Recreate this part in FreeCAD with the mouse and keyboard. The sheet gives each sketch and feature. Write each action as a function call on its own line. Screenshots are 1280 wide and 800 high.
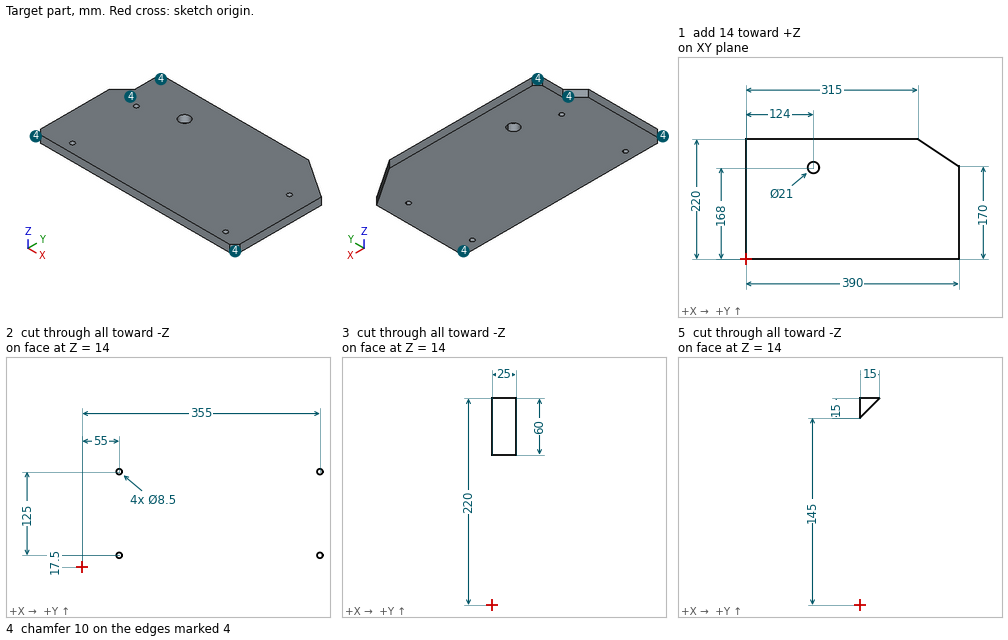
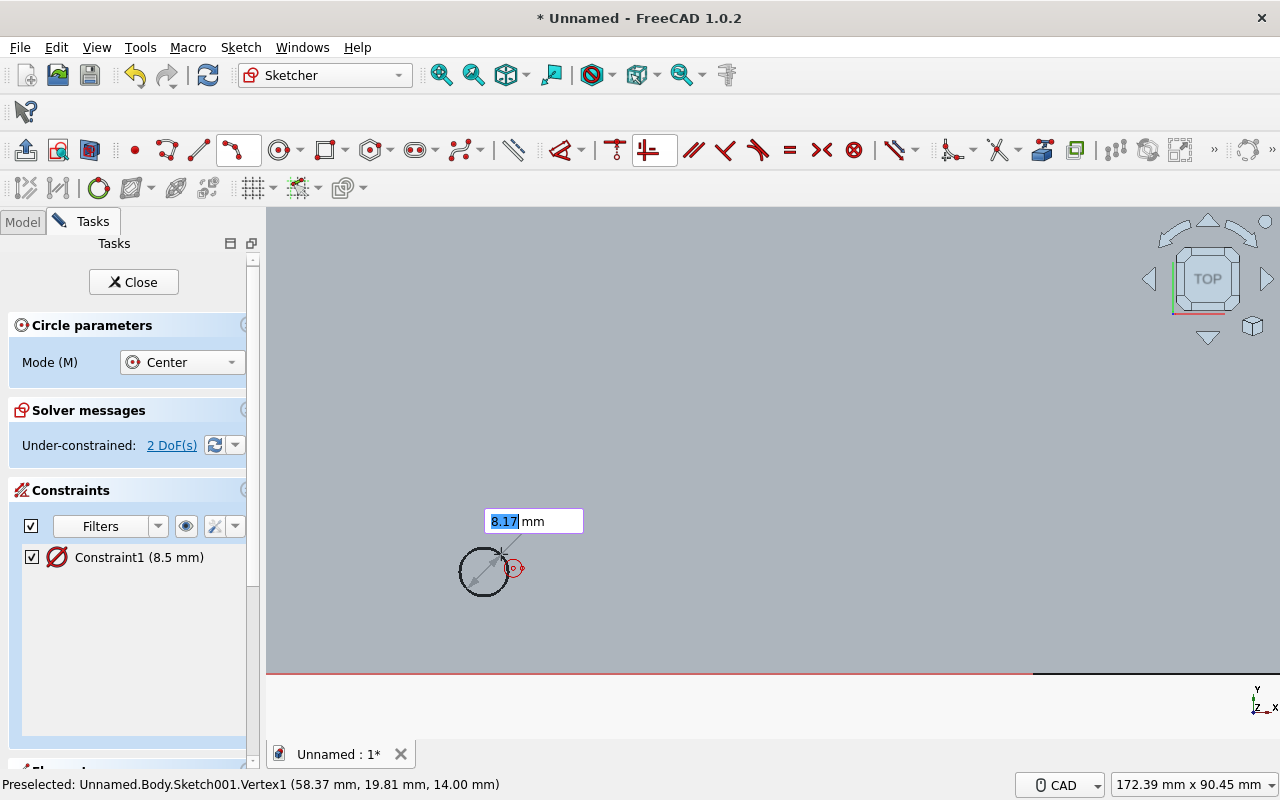
text(8.5)
key(Return)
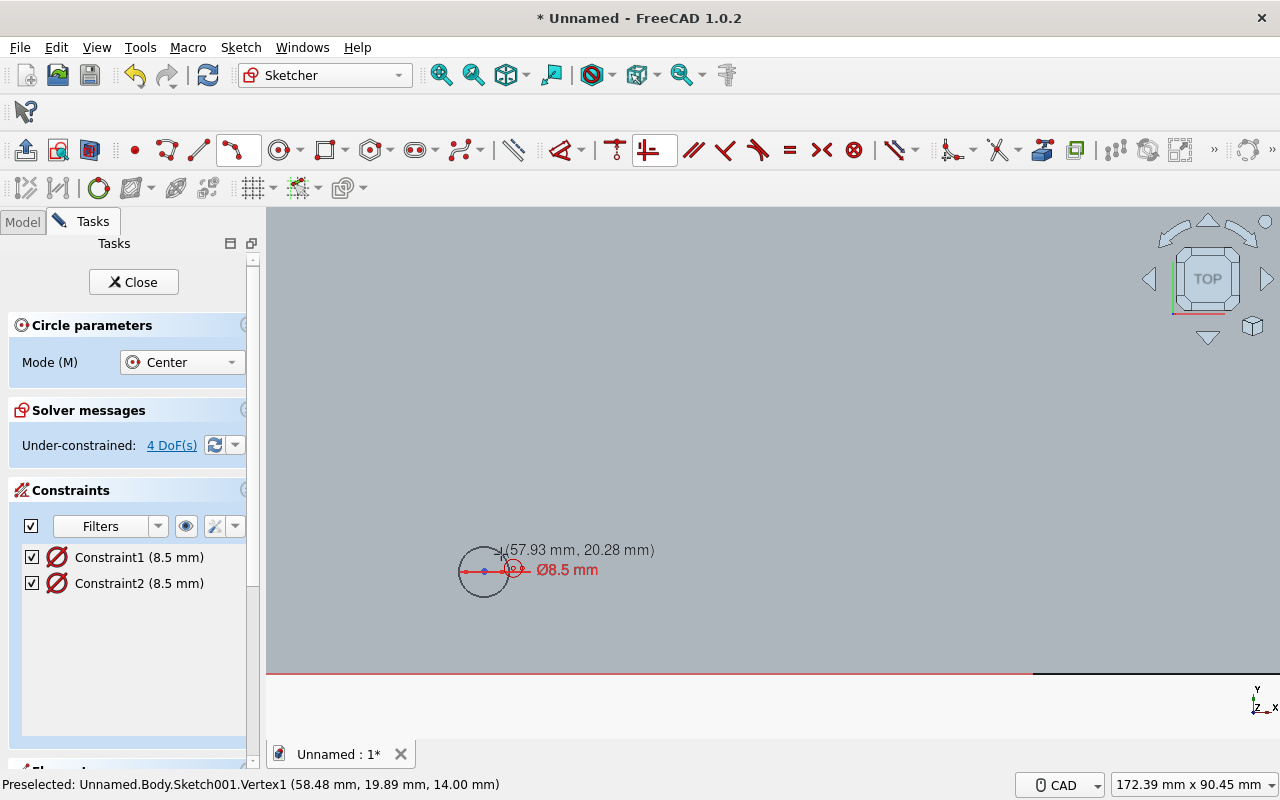
scroll(484, 572, down, 6)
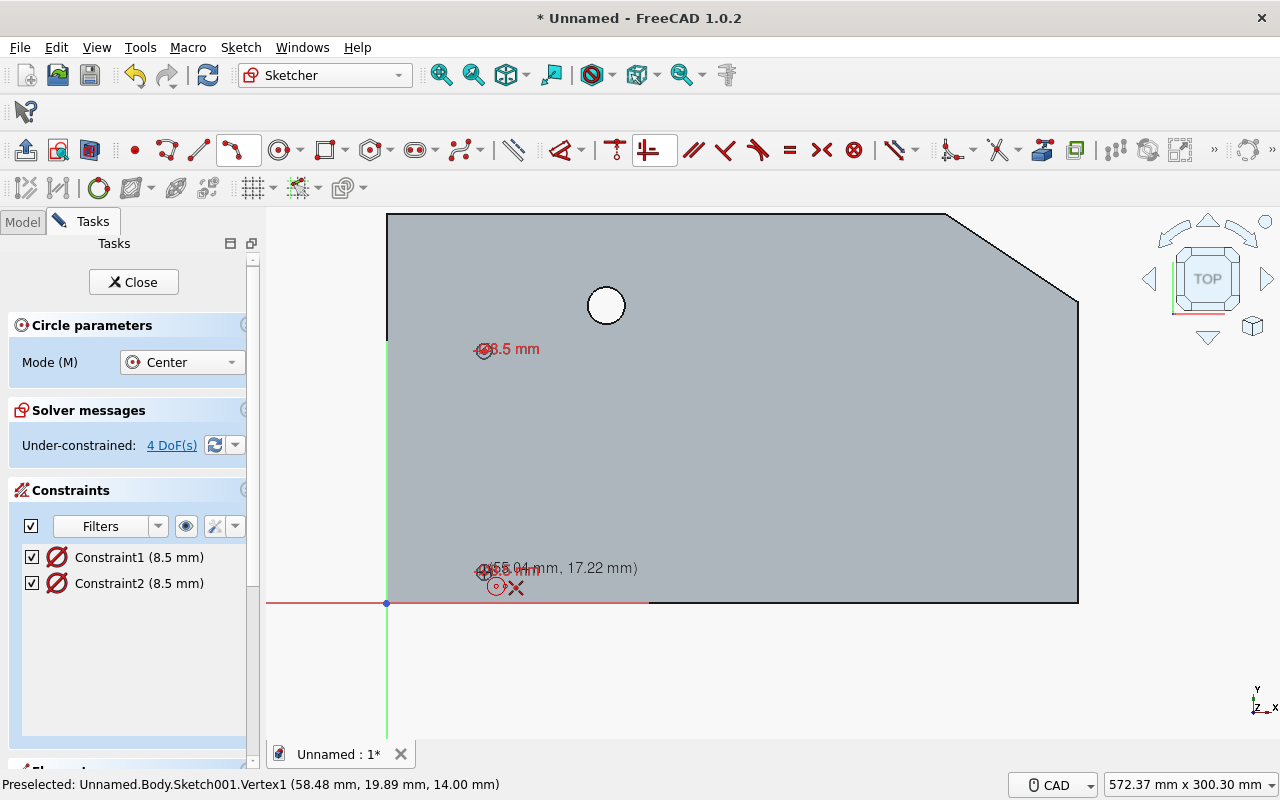
scroll(1016, 351, up, 6)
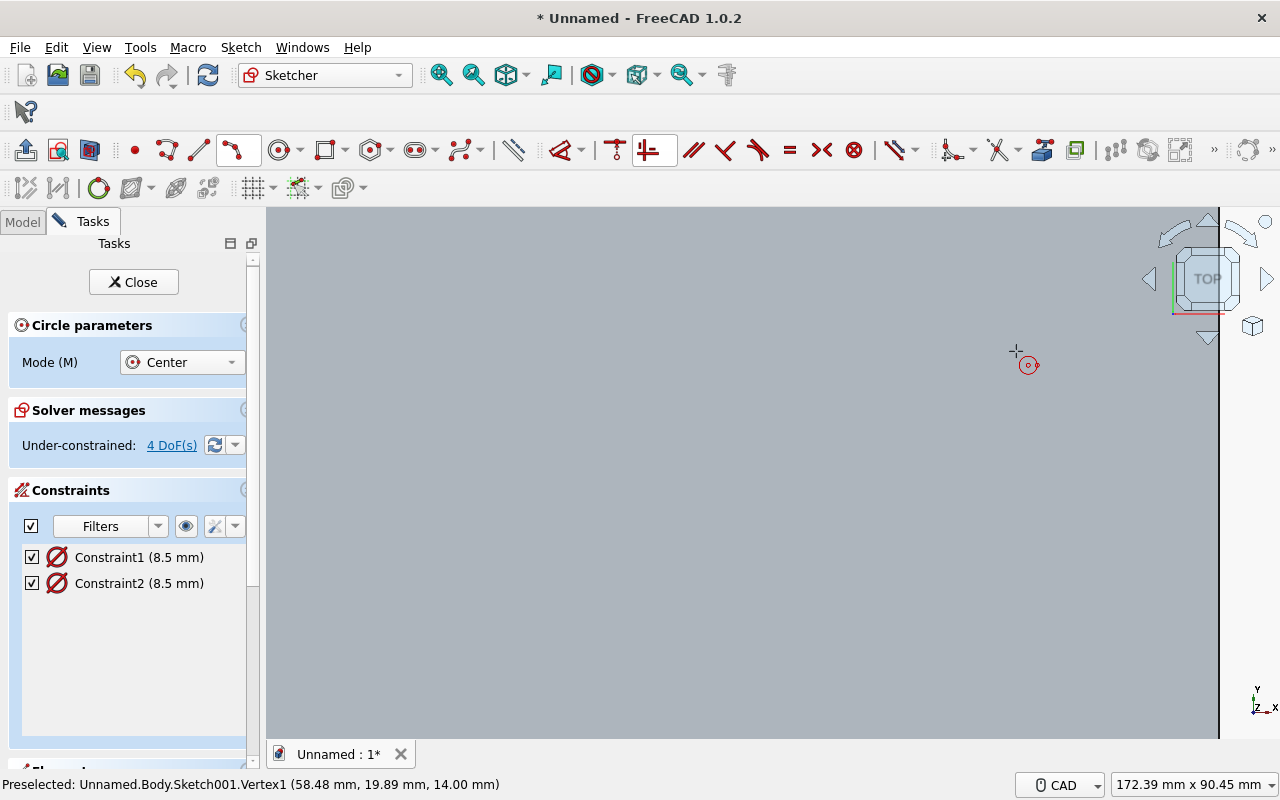
click(1013, 350)
move(1030, 332)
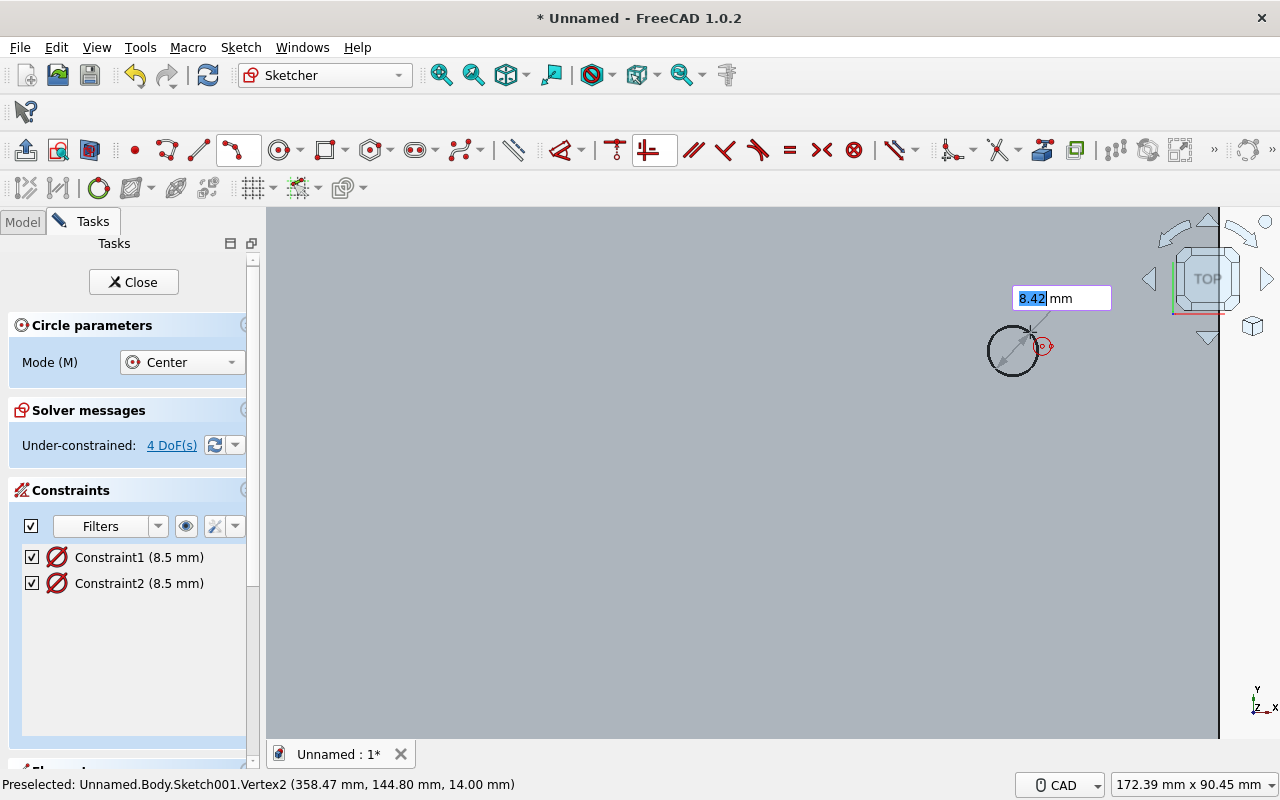
text(8.5)
key(Return)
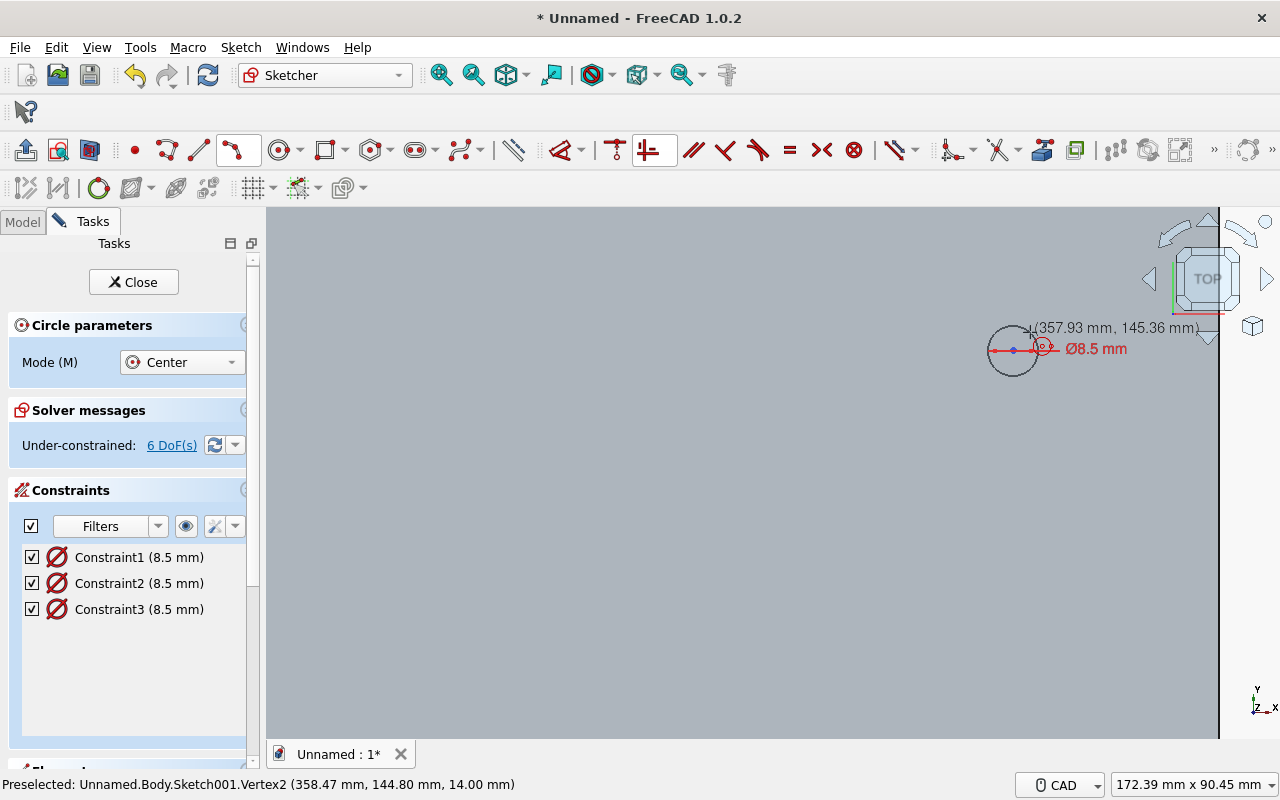
scroll(1016, 351, down, 6)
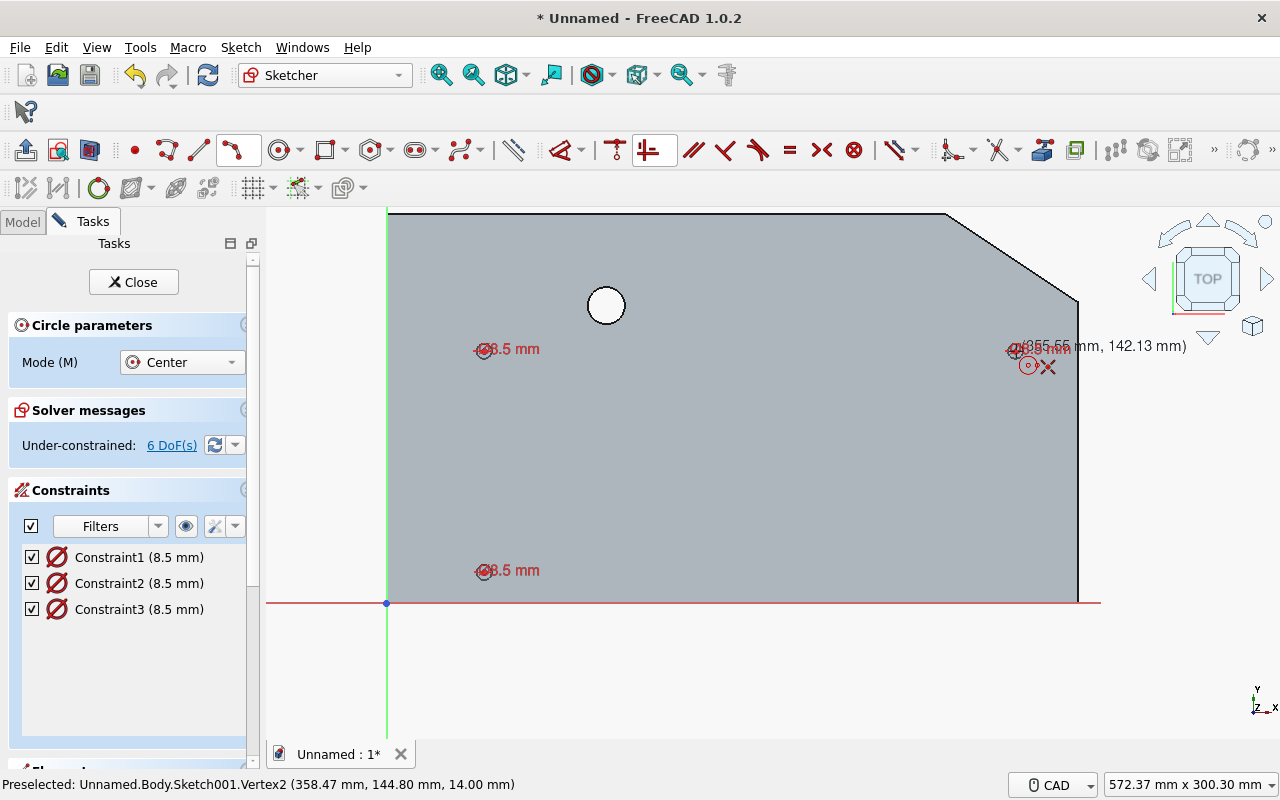
scroll(1016, 572, up, 6)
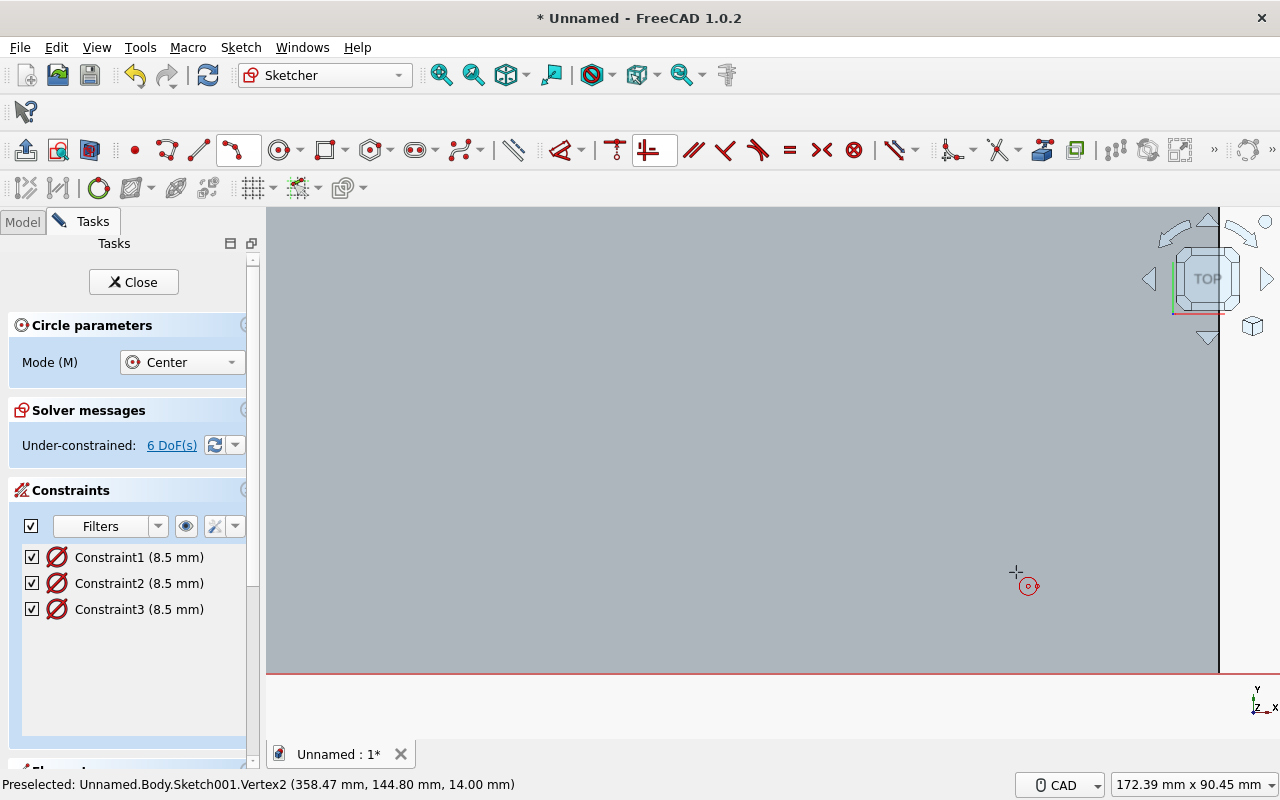
click(1013, 571)
move(1030, 554)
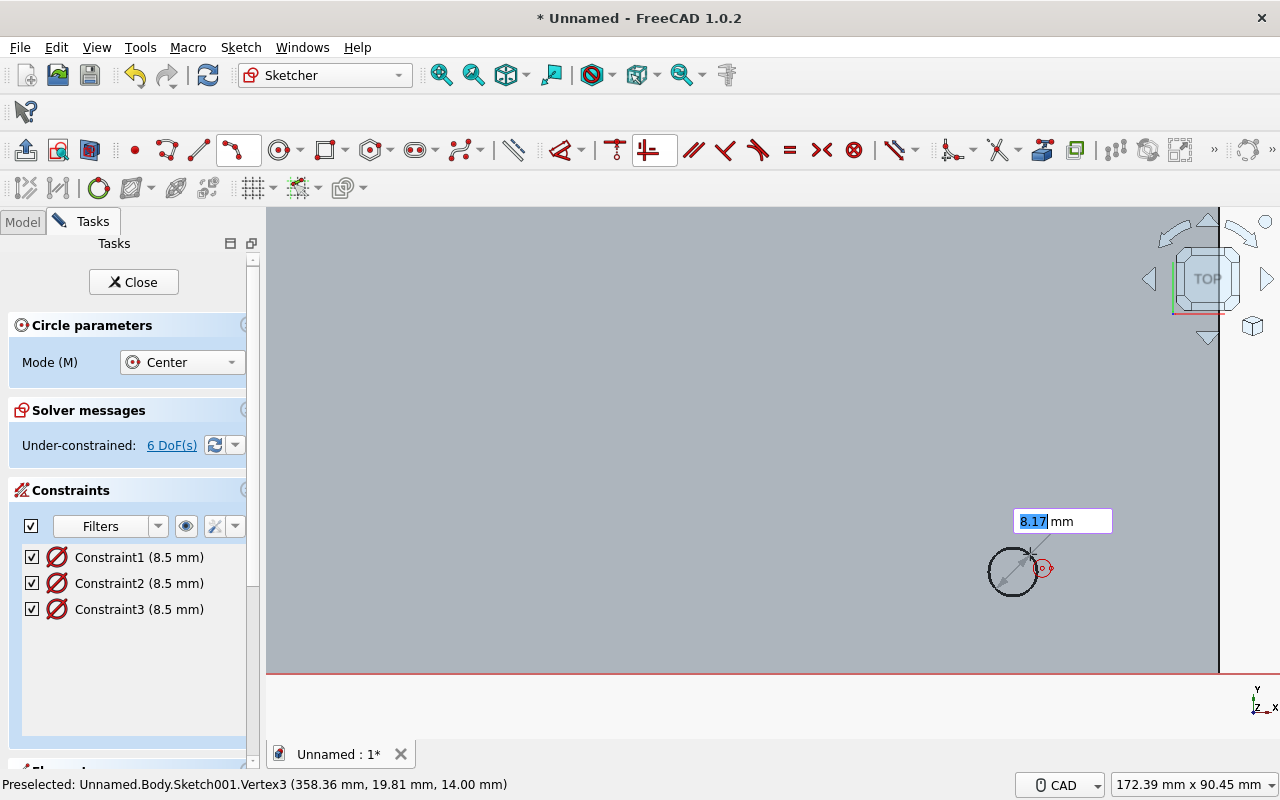
text(8.5)
key(Return)
key(Escape)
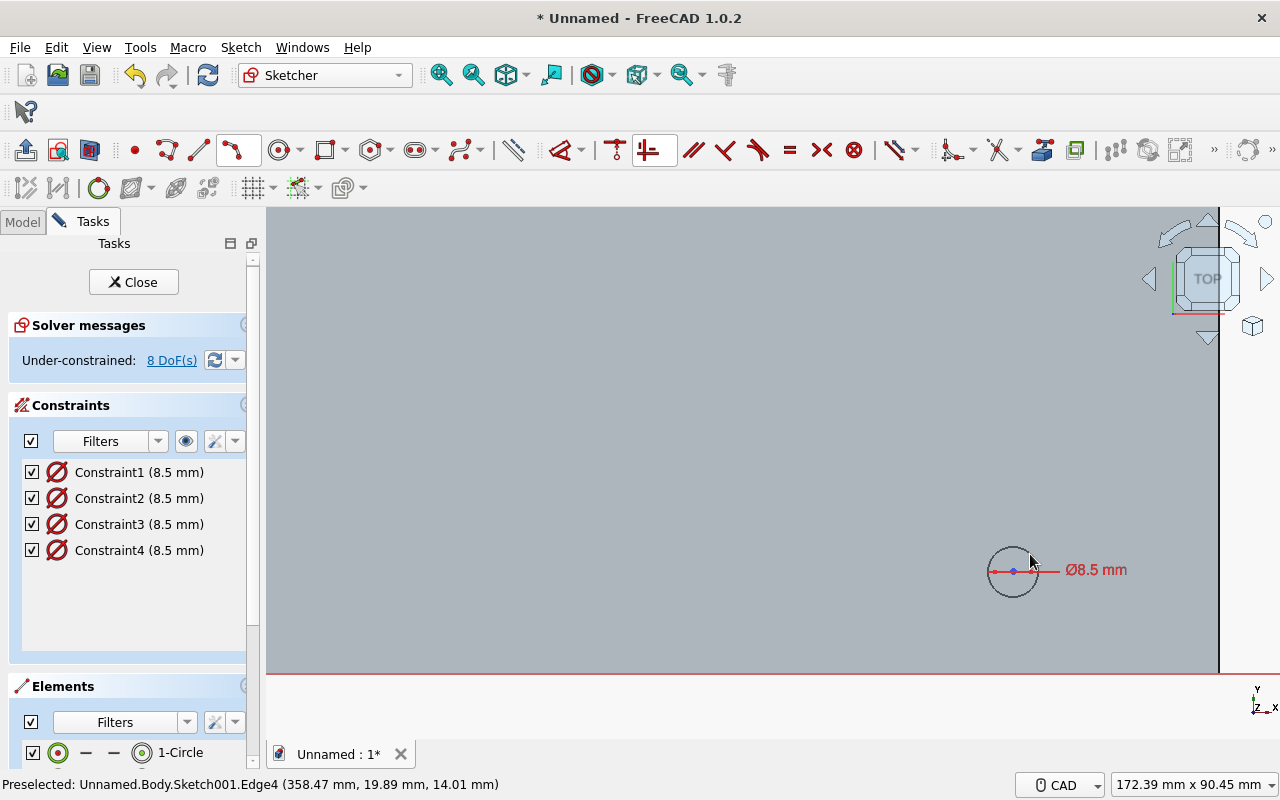
scroll(1016, 572, down, 6)